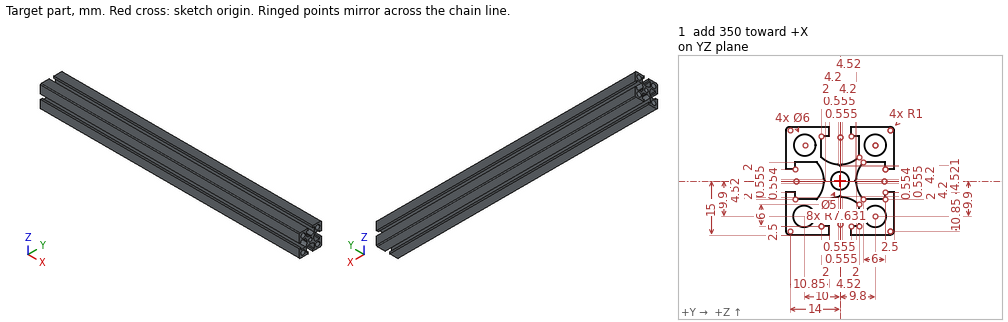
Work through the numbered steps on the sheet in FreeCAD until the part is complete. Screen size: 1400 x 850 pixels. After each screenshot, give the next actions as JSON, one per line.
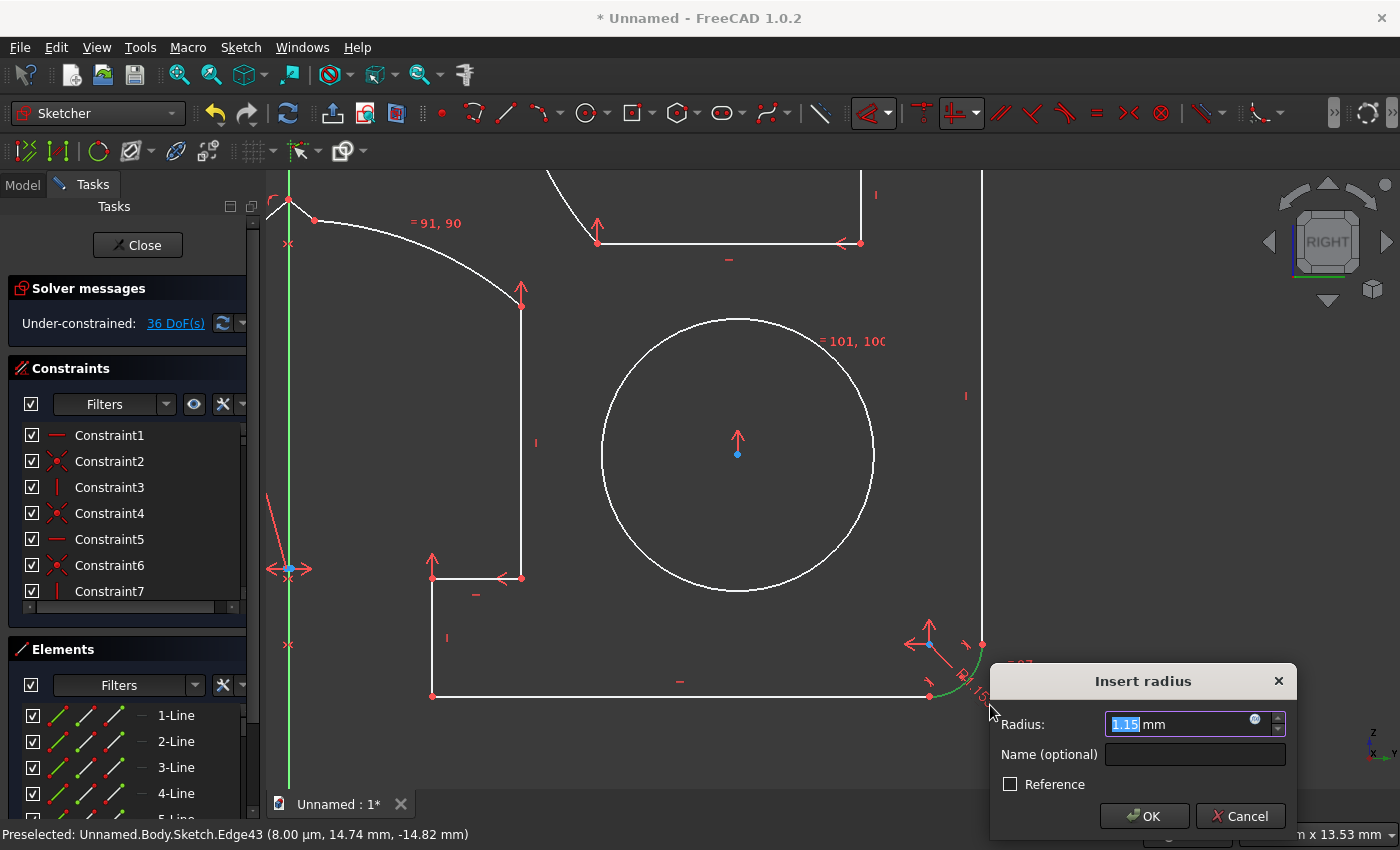
{"action": "type", "text": "1"}
{"action": "key", "text": "Return"}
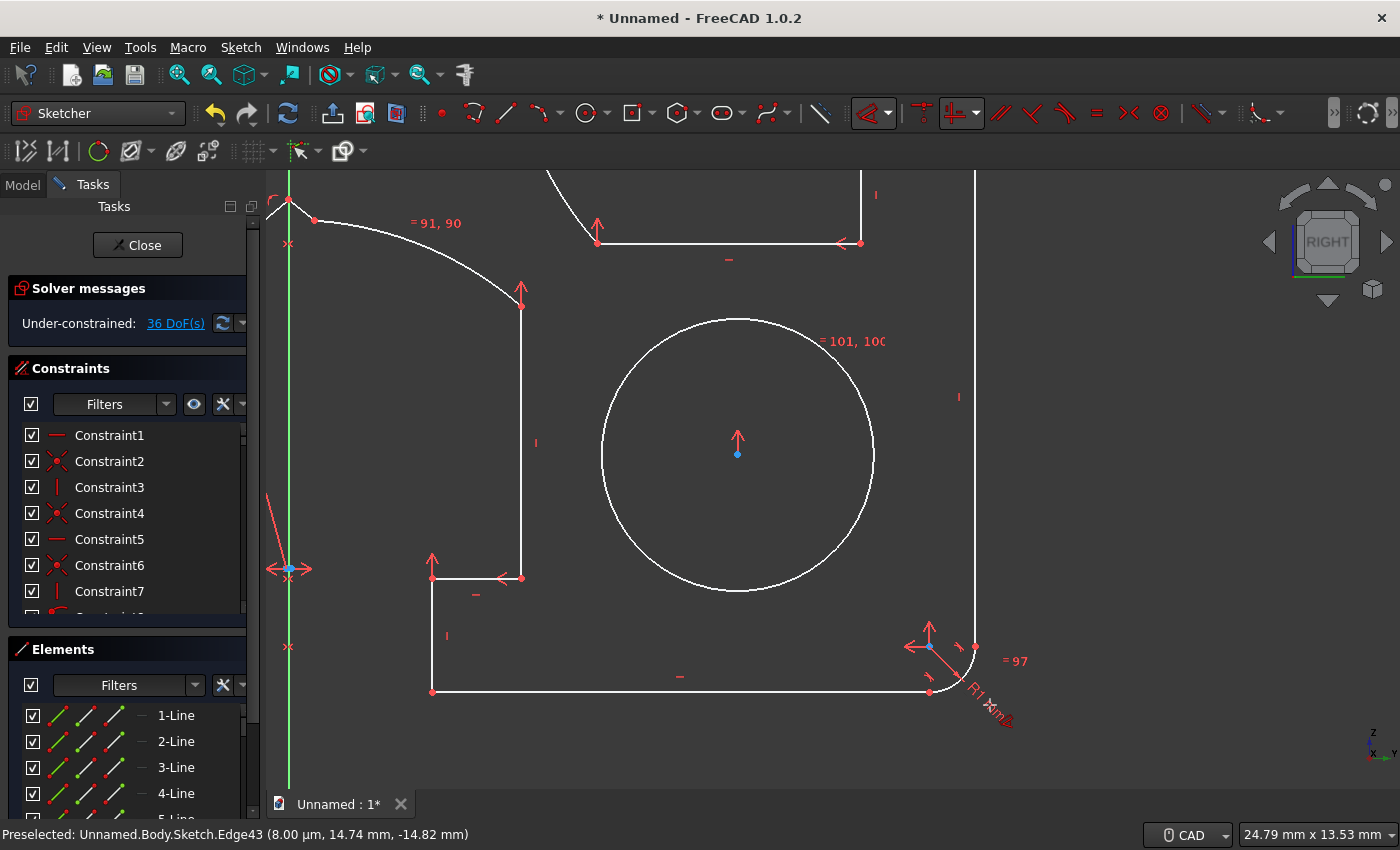
{"action": "scroll", "coordinate": [969, 683], "scroll_direction": "down", "scroll_amount": 6}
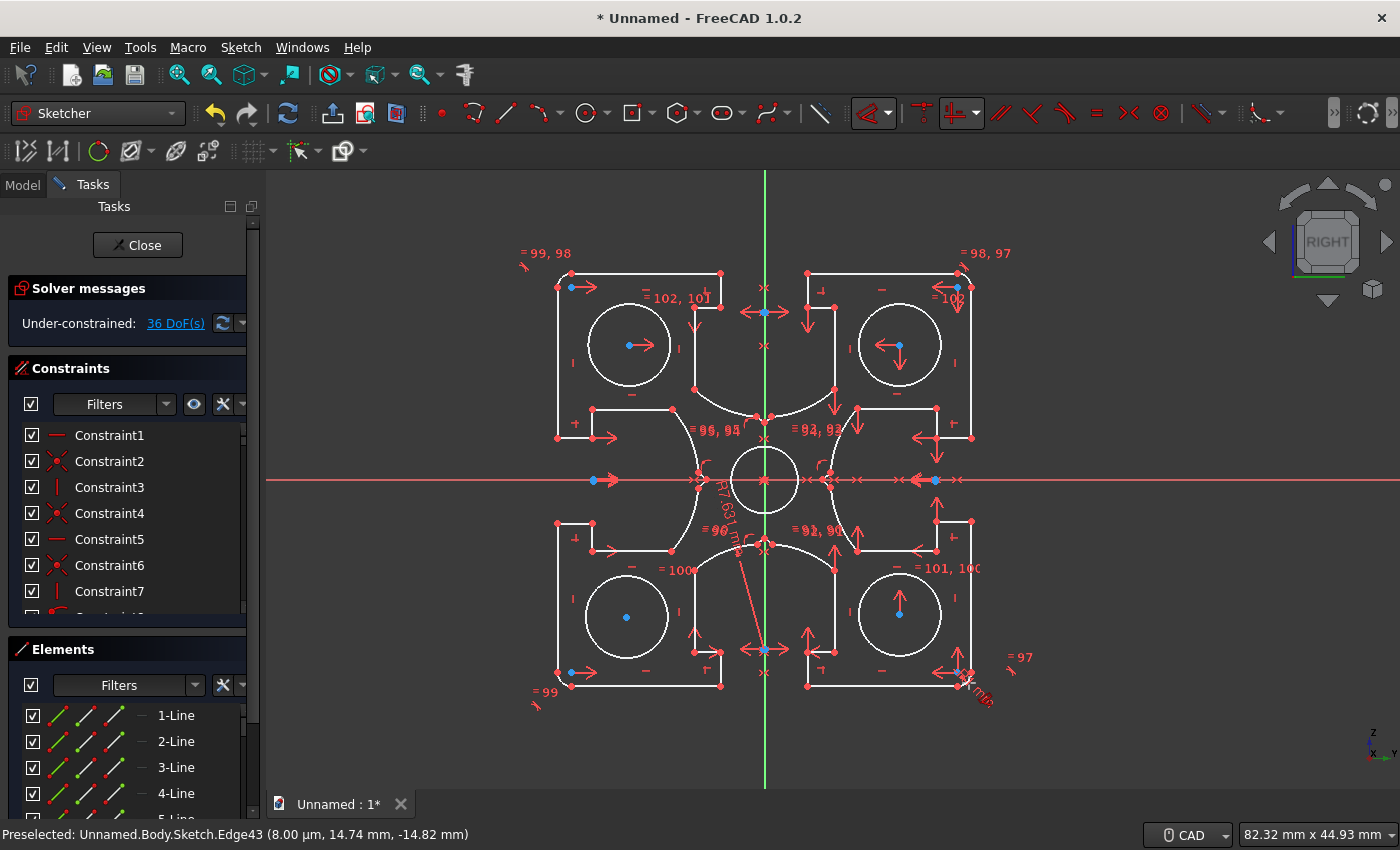
{"action": "left_click", "coordinate": [656, 588]}
{"action": "left_click", "coordinate": [679, 565]}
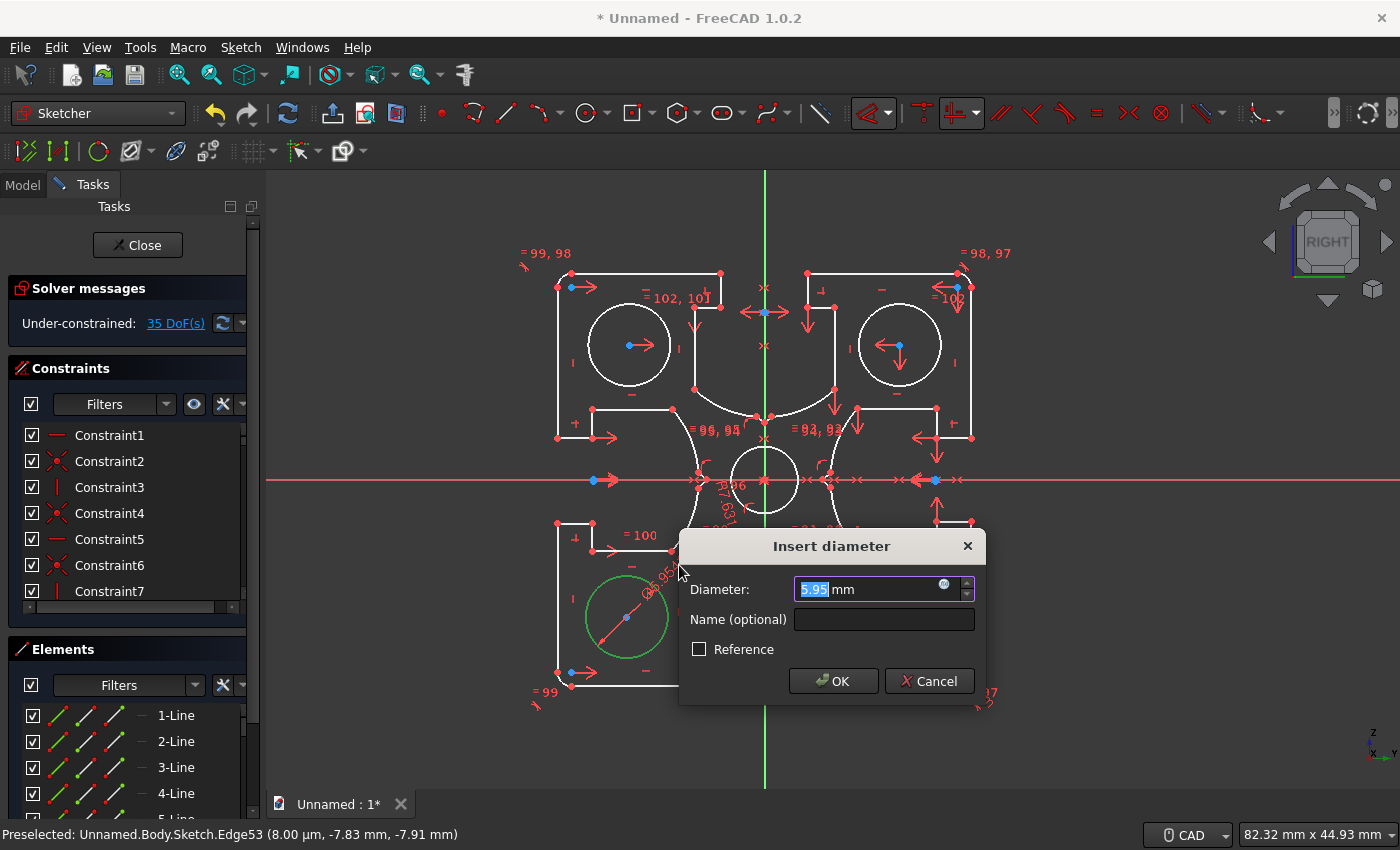
{"action": "type", "text": "6"}
{"action": "key", "text": "Return"}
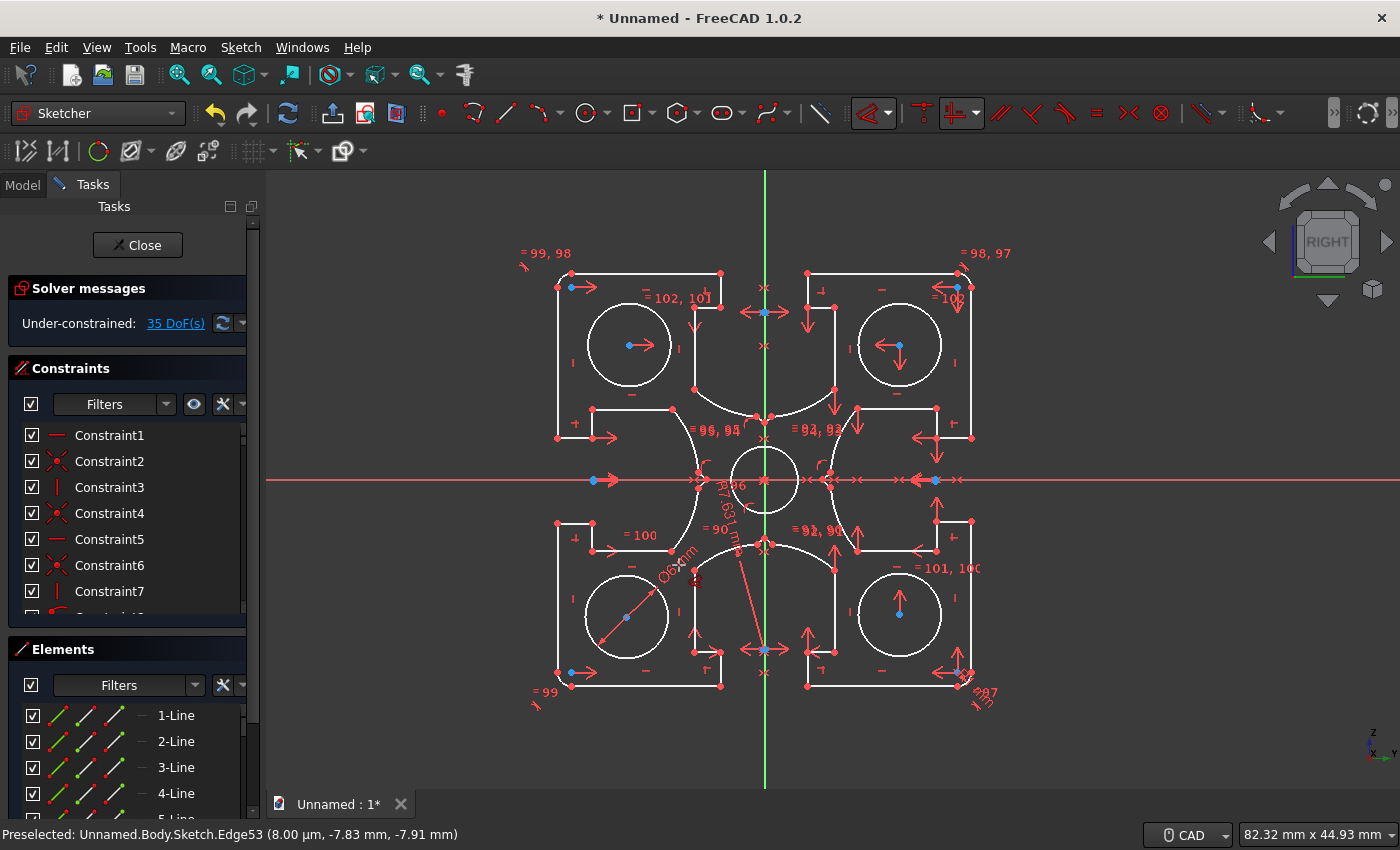
{"action": "left_click", "coordinate": [788, 456]}
{"action": "left_click", "coordinate": [810, 433]}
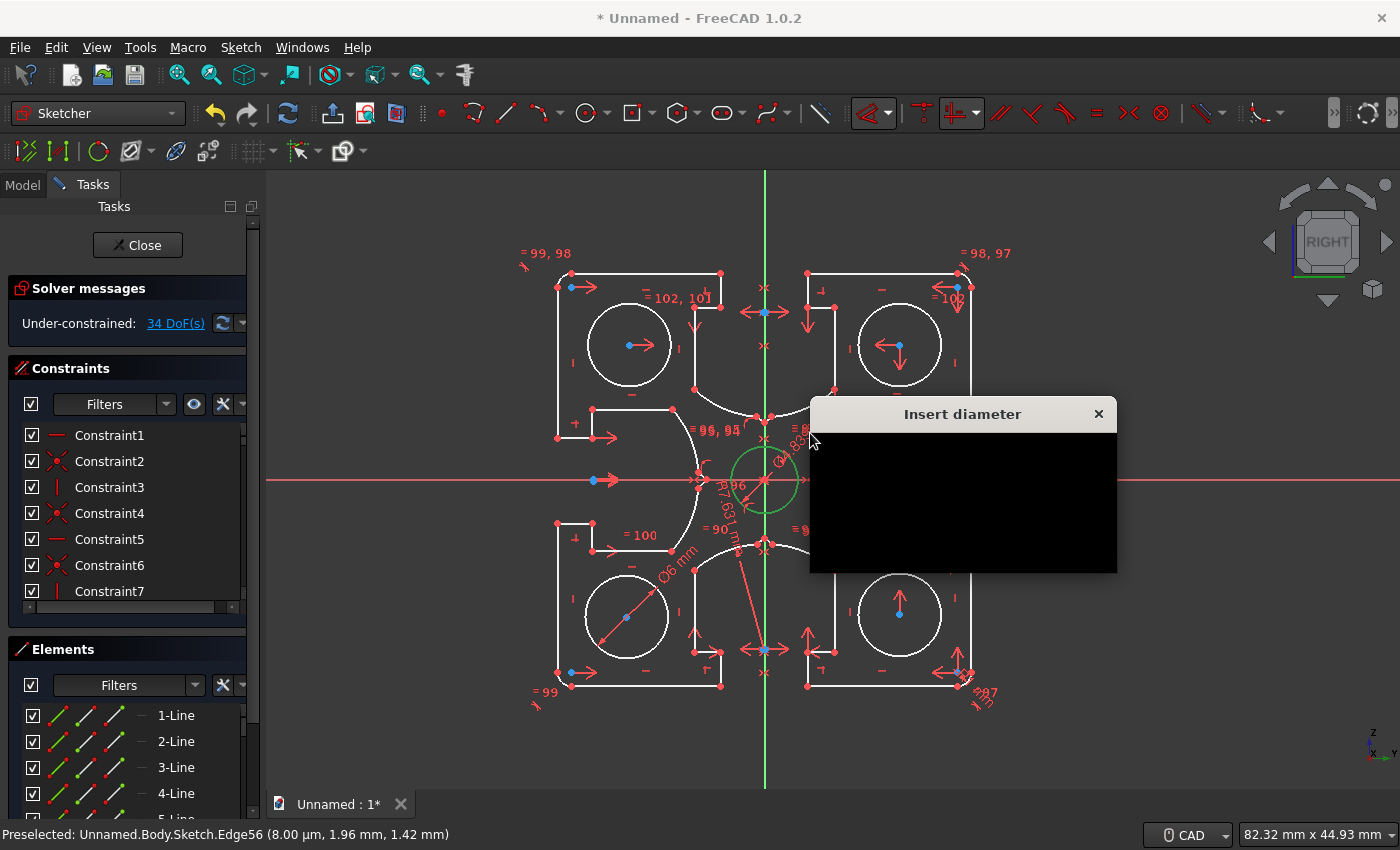
{"action": "type", "text": "5"}
{"action": "key", "text": "Return"}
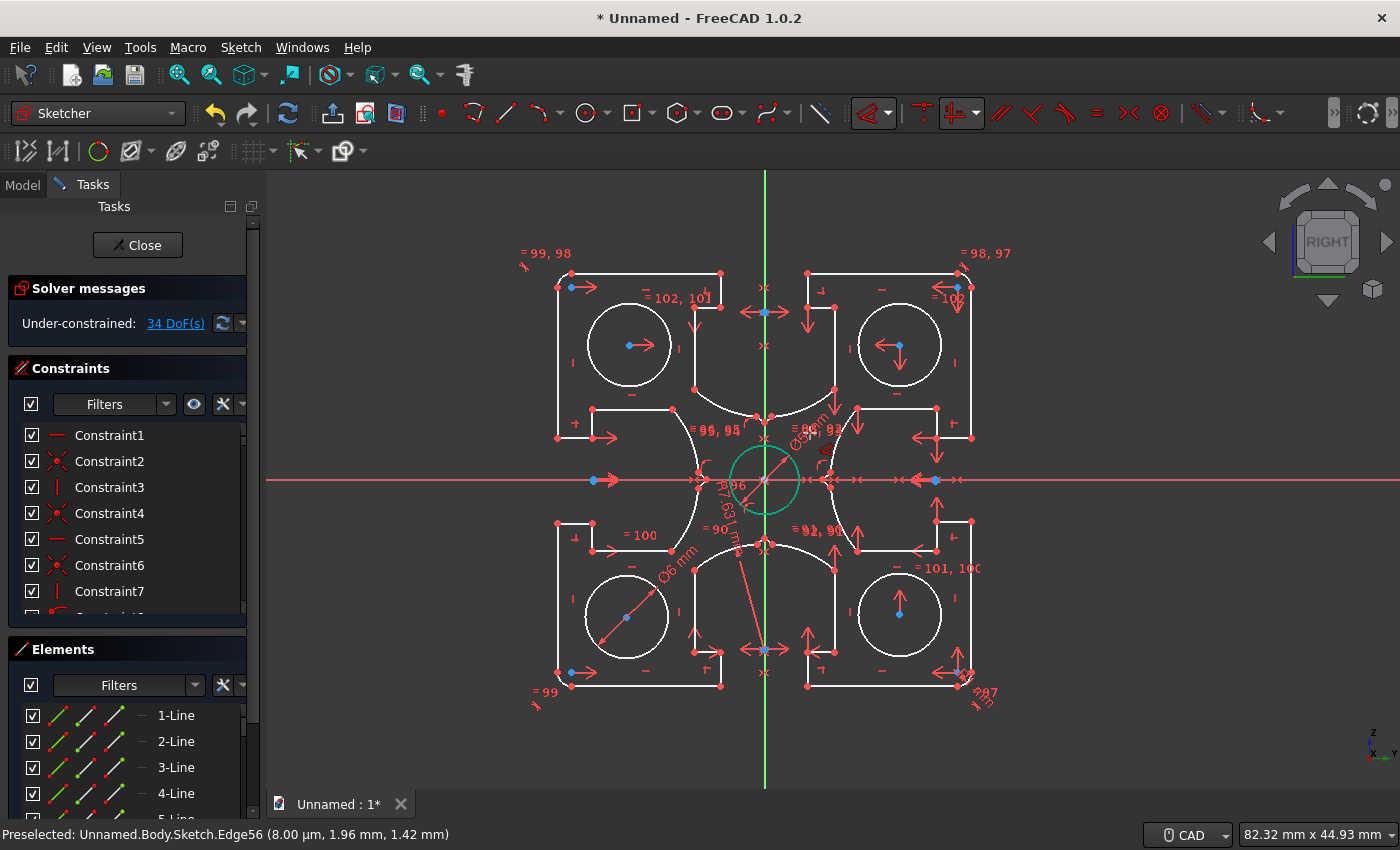
{"action": "scroll", "coordinate": [710, 652], "scroll_direction": "up", "scroll_amount": 2}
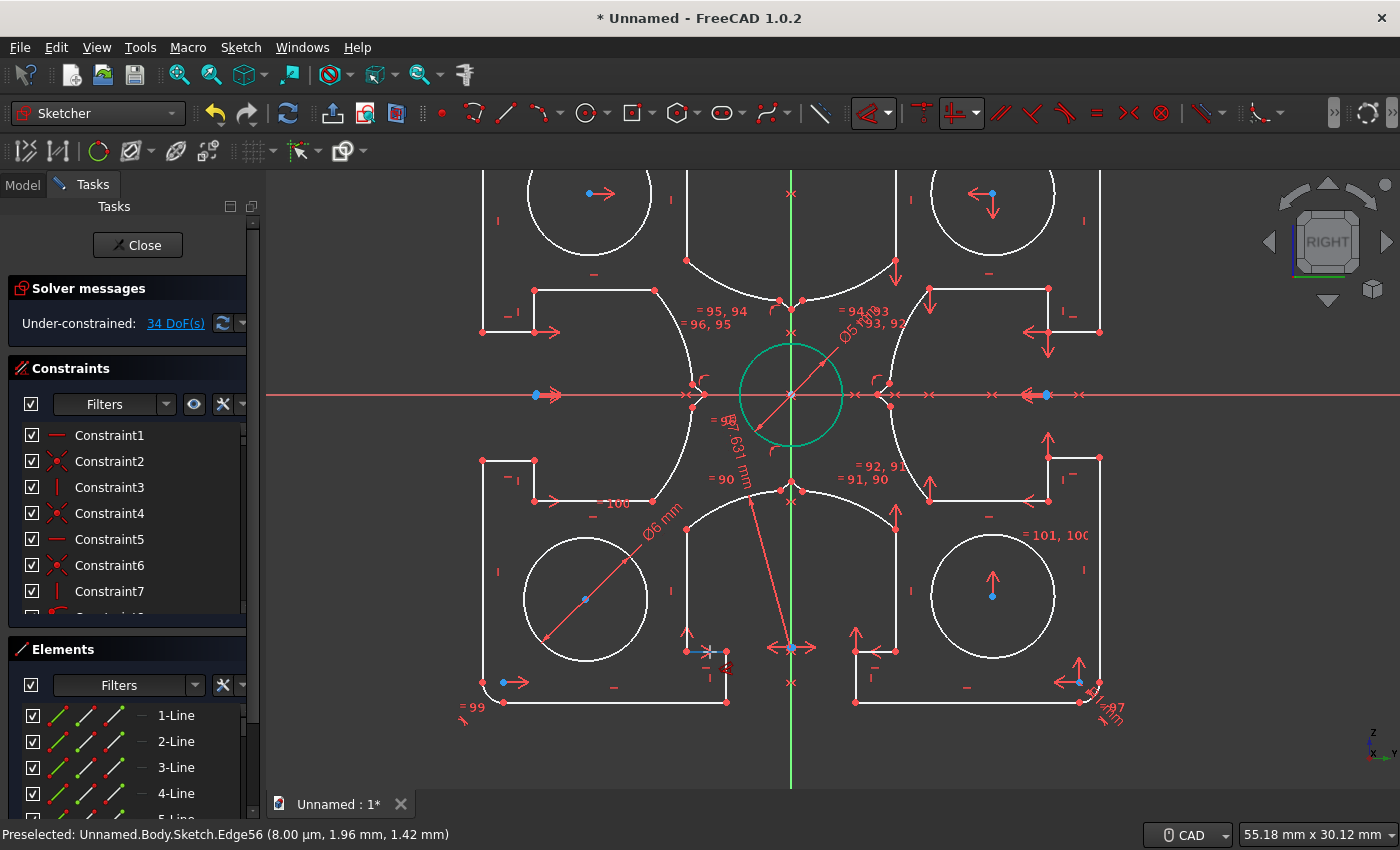
{"action": "left_click", "coordinate": [710, 652]}
{"action": "left_click", "coordinate": [706, 686]}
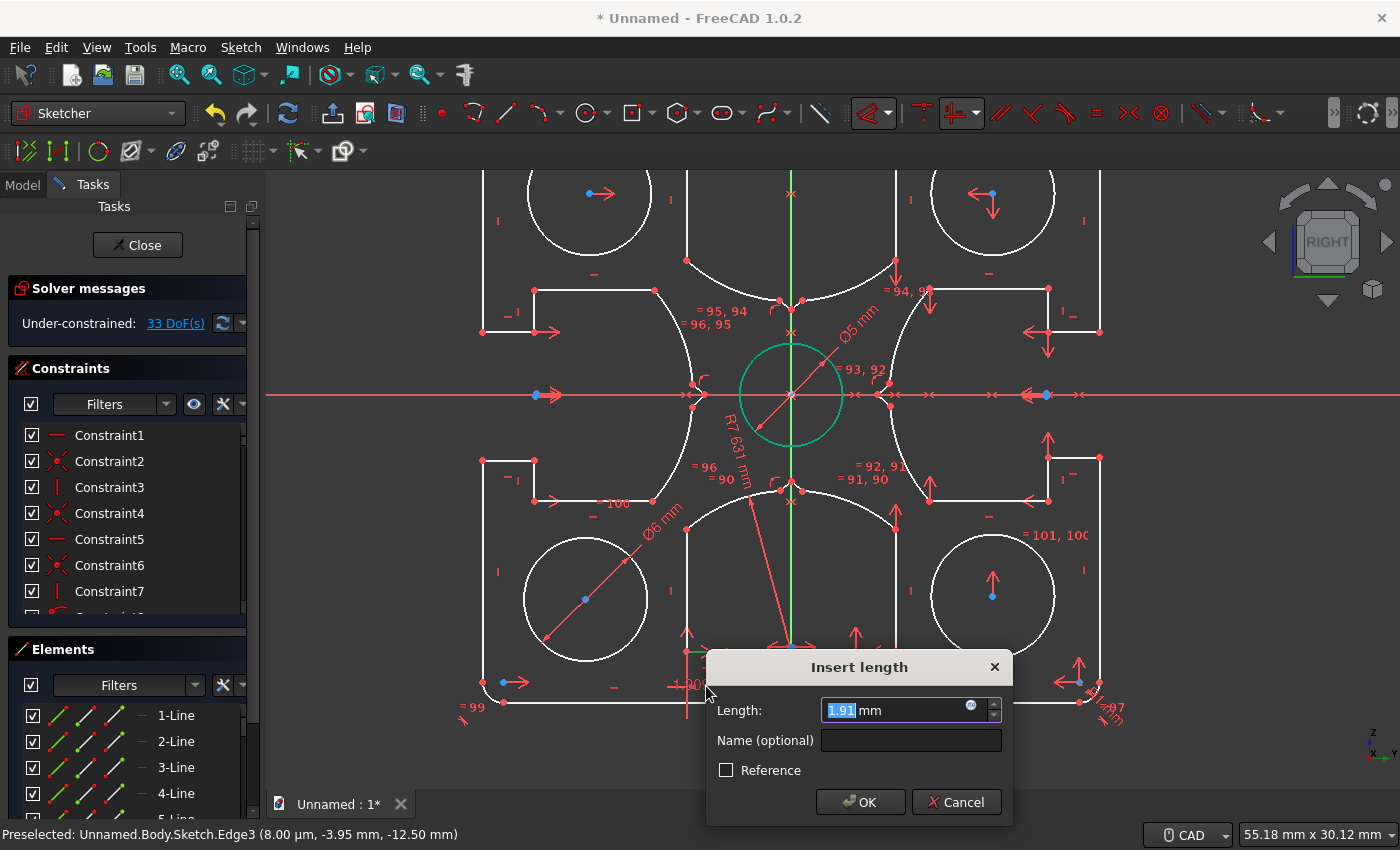
{"action": "type", "text": "2"}
{"action": "key", "text": "Return"}